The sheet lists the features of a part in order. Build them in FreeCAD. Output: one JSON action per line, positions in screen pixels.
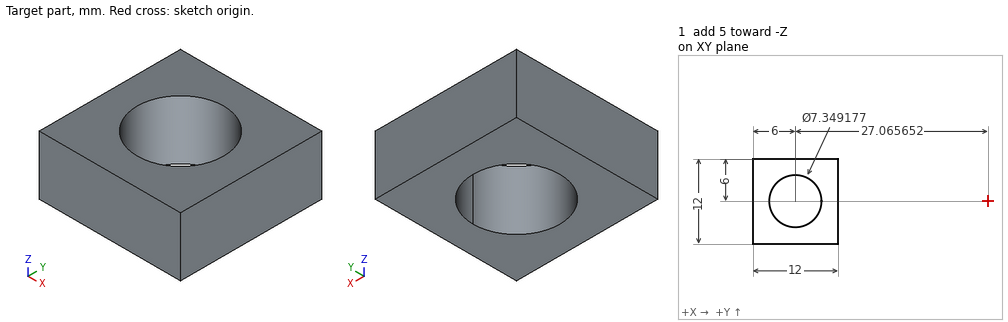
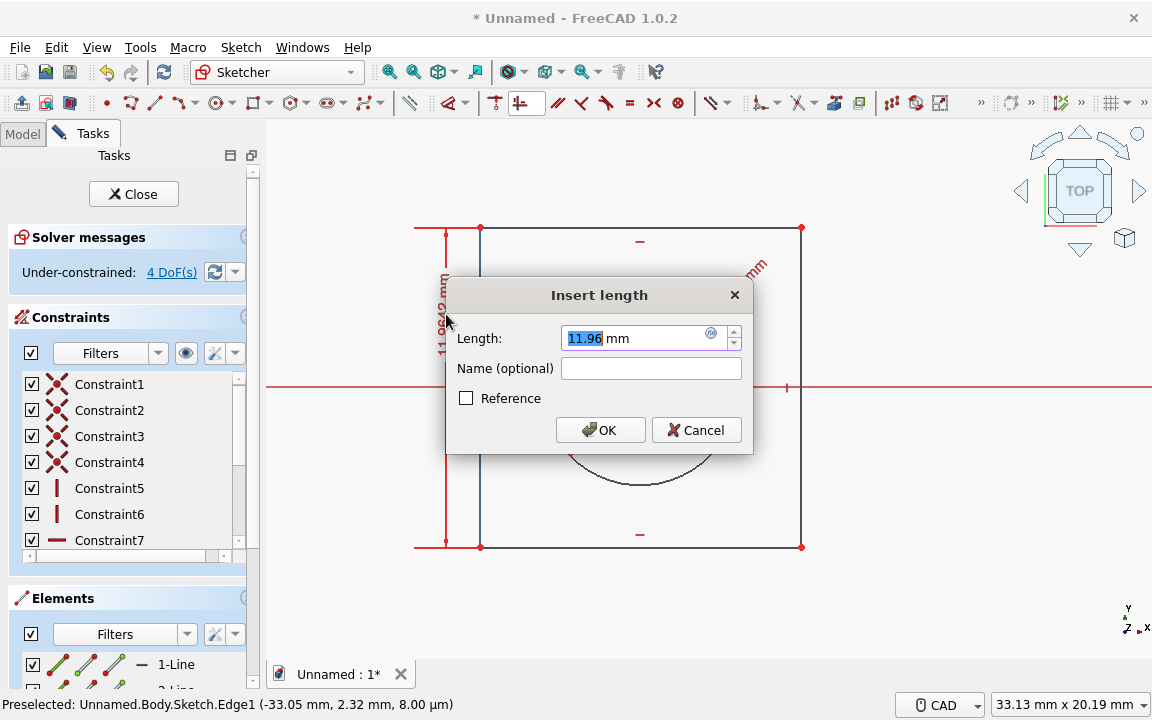
{"action": "type", "text": "12"}
{"action": "key", "text": "Return"}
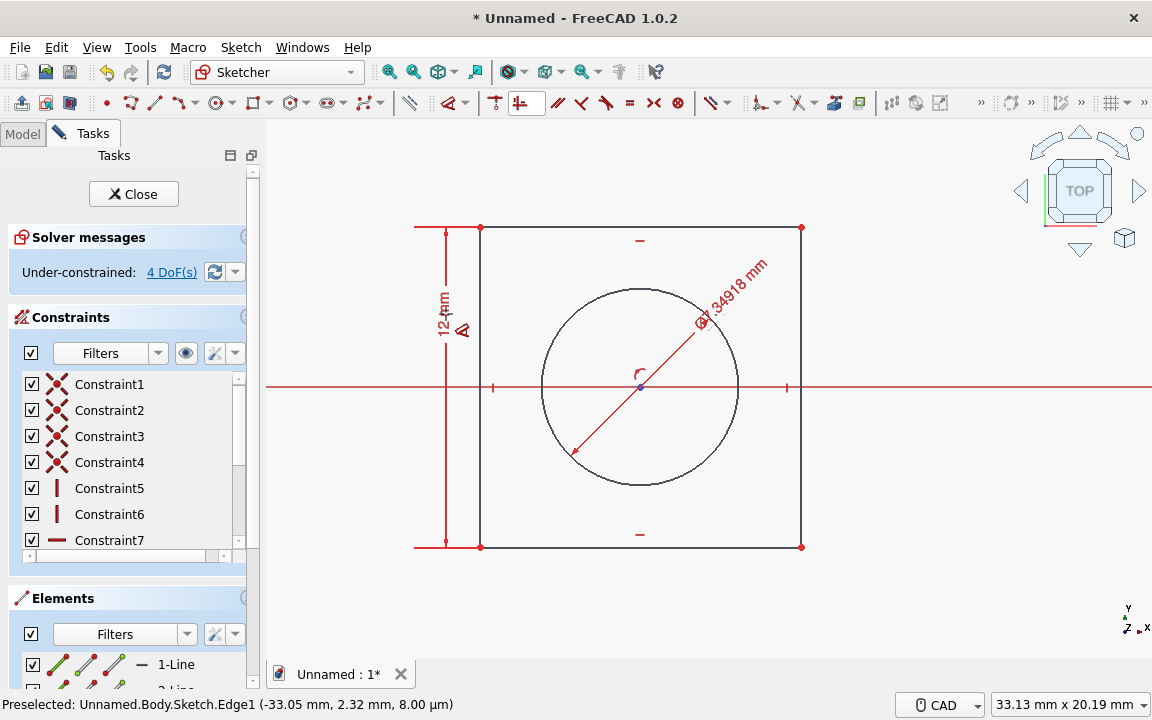
{"action": "left_click", "coordinate": [576, 548]}
{"action": "left_click", "coordinate": [641, 582]}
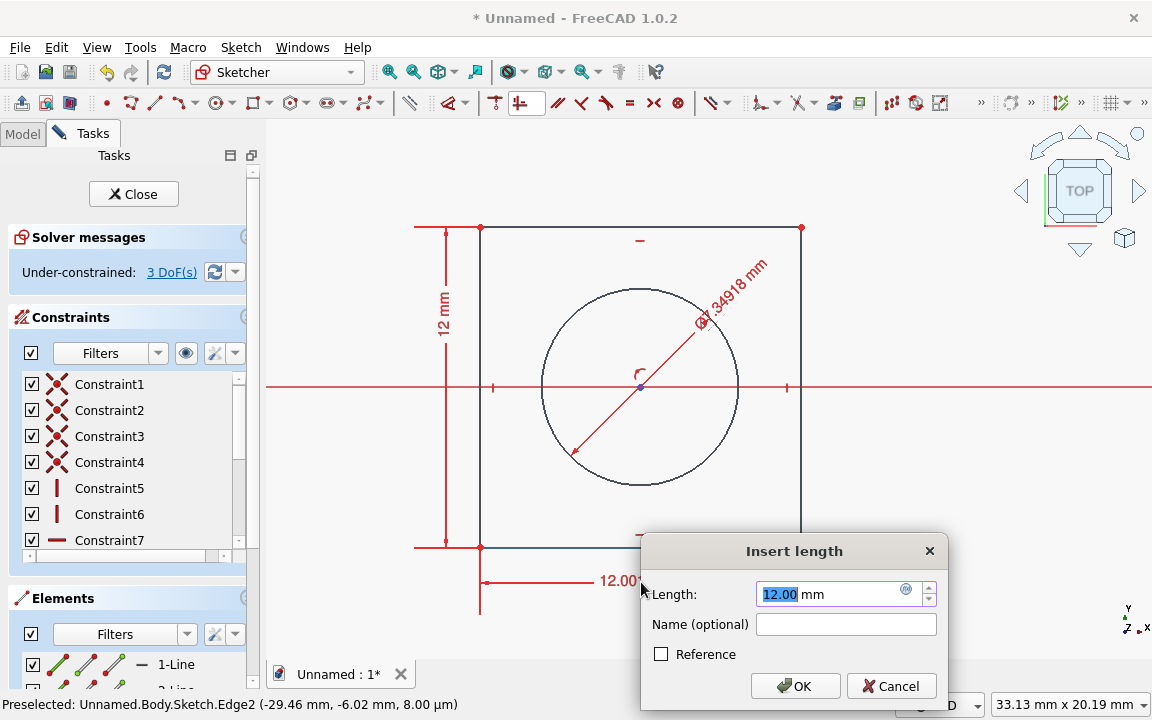
{"action": "type", "text": "12"}
{"action": "key", "text": "Return"}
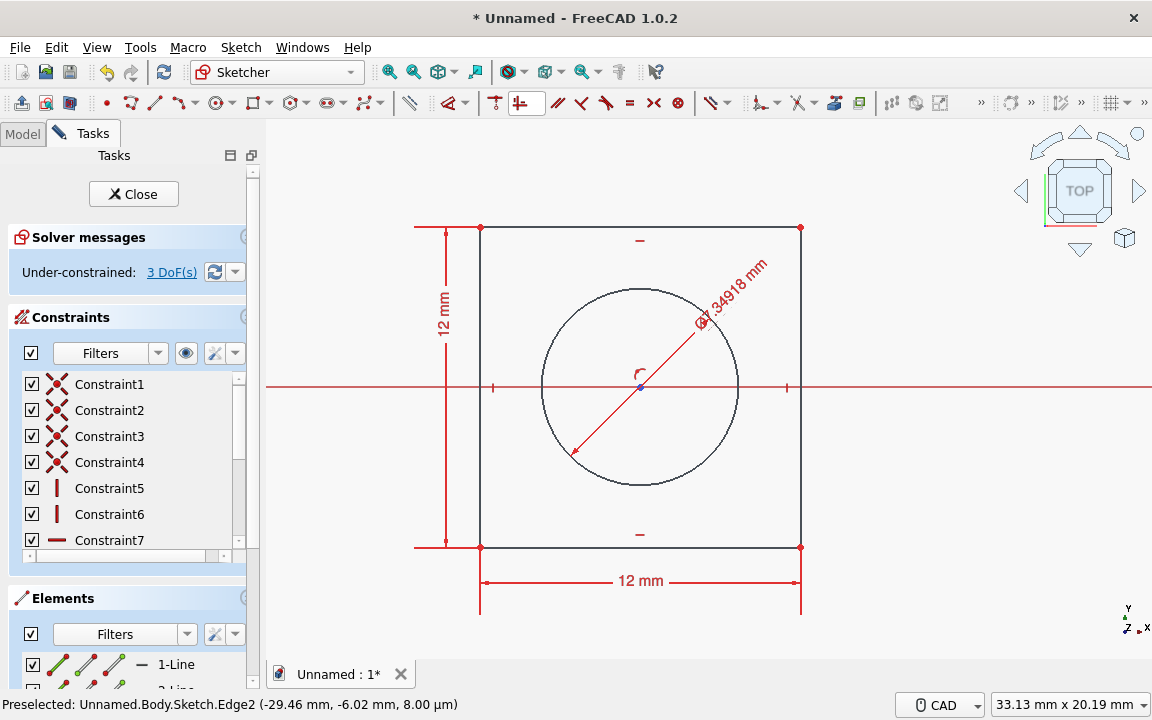
{"action": "left_click", "coordinate": [480, 227]}
{"action": "left_click", "coordinate": [446, 270]}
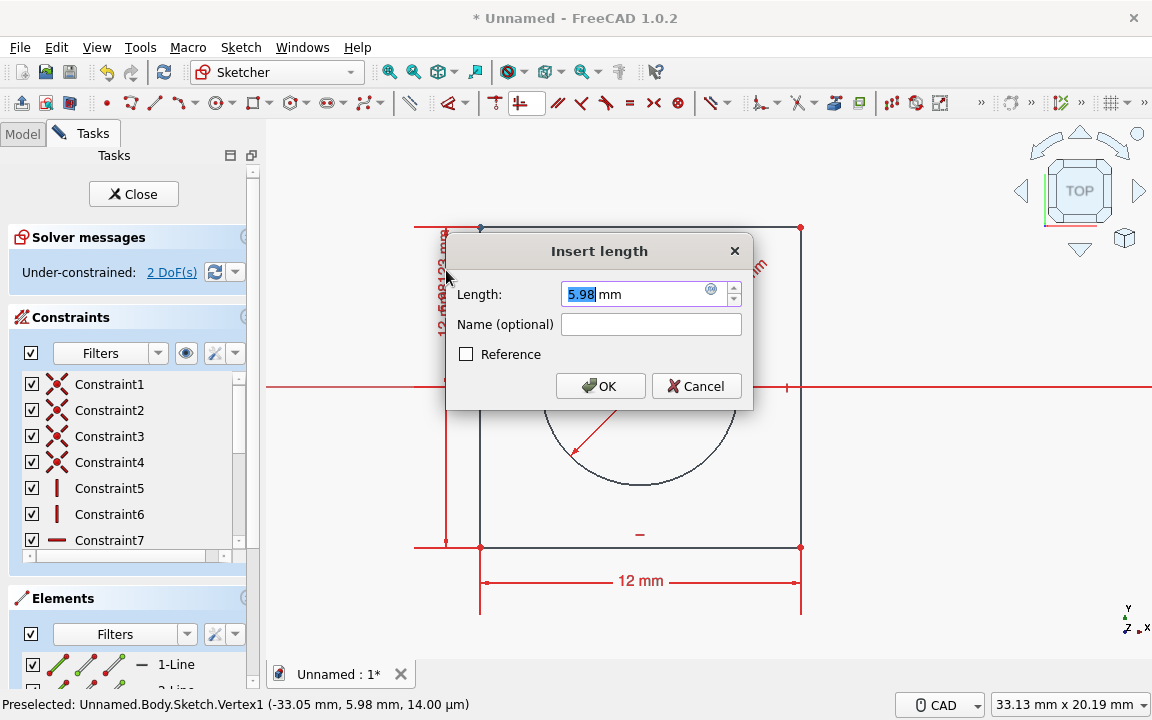
{"action": "type", "text": "6"}
{"action": "key", "text": "Return"}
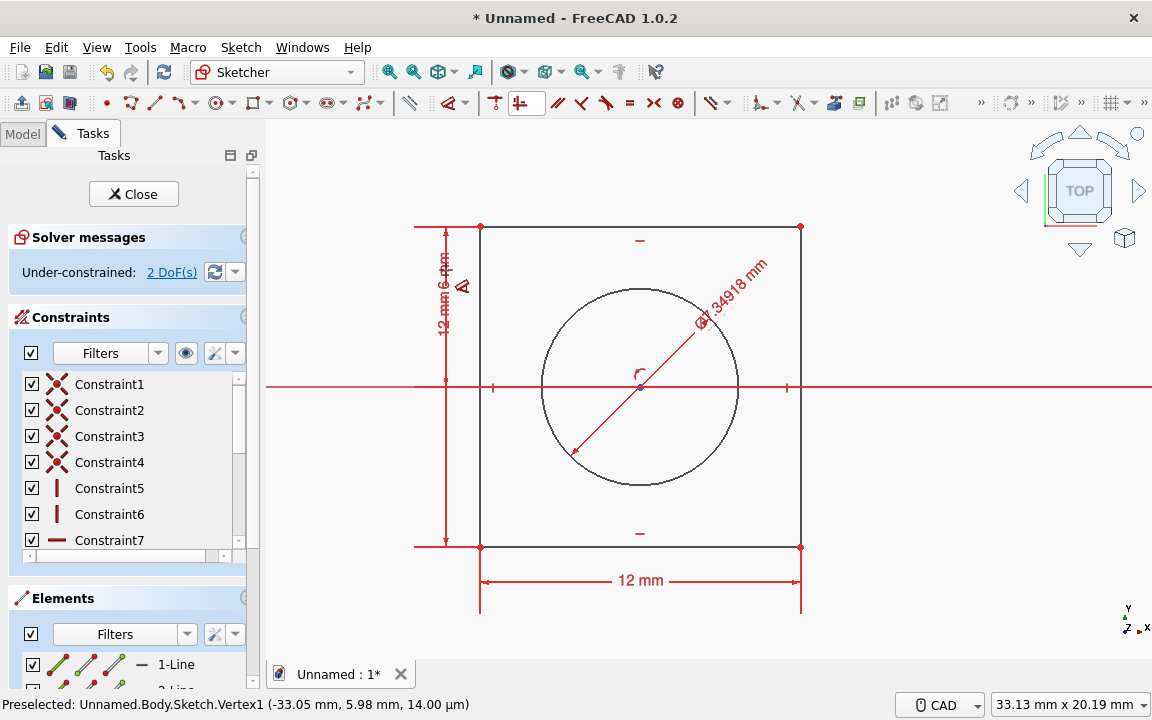
{"action": "left_click", "coordinate": [480, 227]}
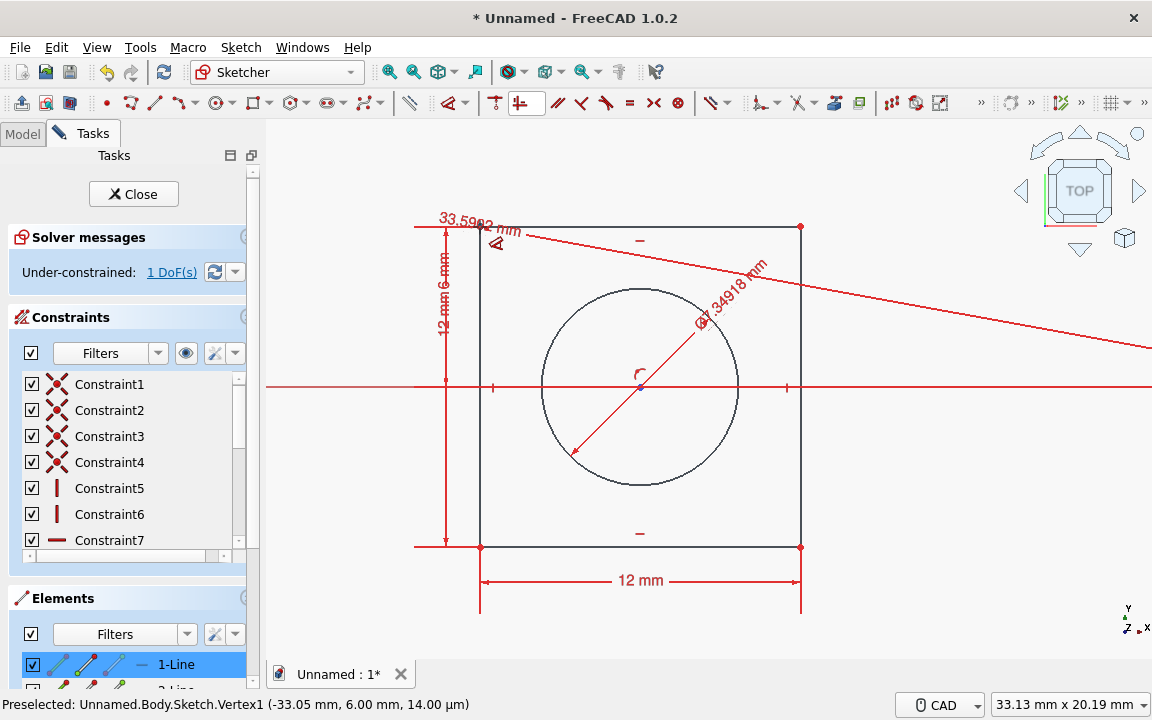
{"action": "left_click", "coordinate": [640, 387]}
{"action": "left_click", "coordinate": [560, 193]}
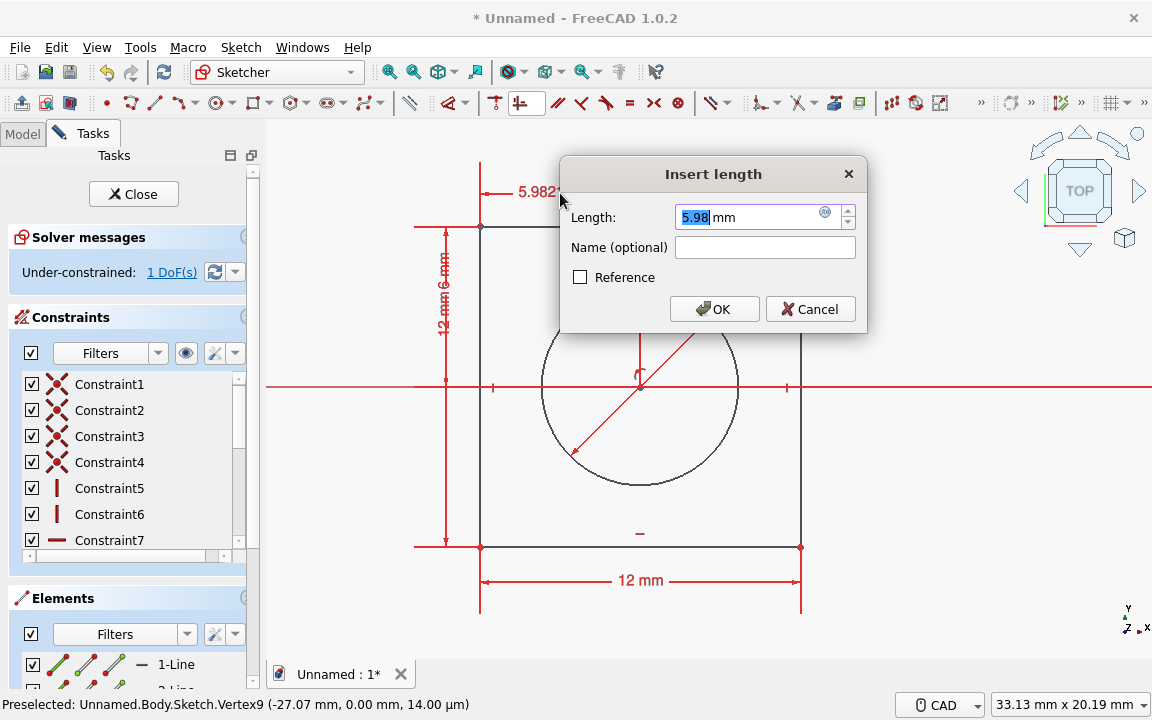
{"action": "type", "text": "6"}
{"action": "key", "text": "Return"}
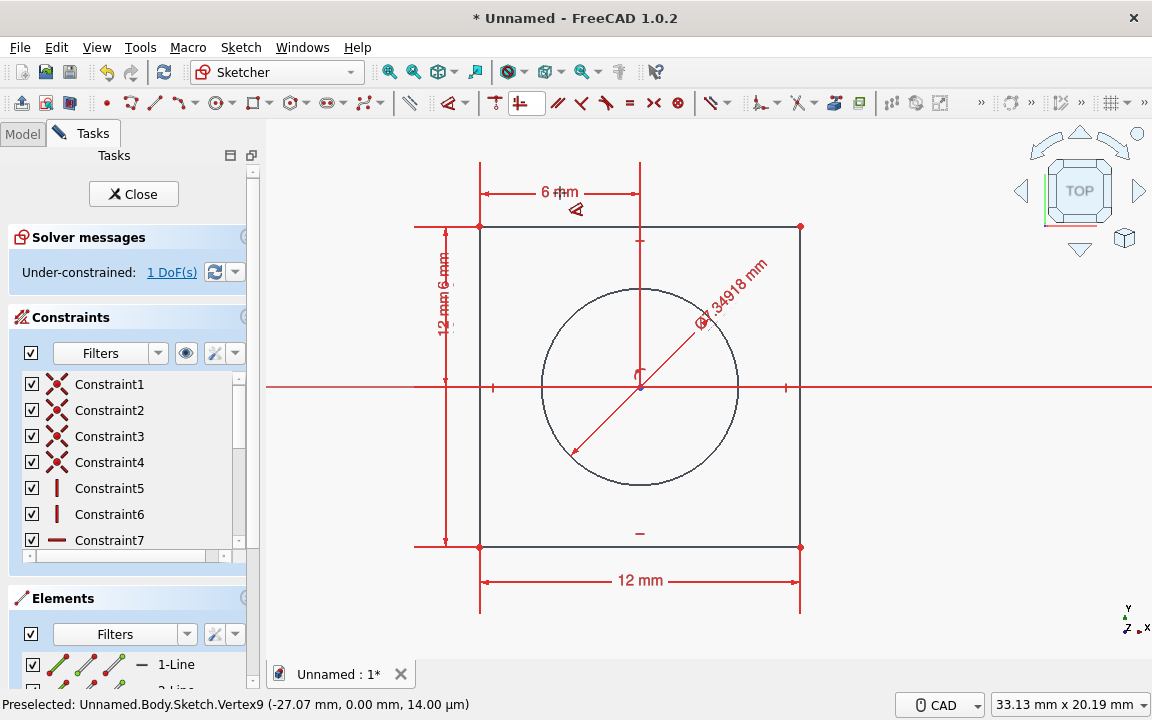
{"action": "left_click", "coordinate": [640, 387]}
{"action": "left_click", "coordinate": [813, 421]}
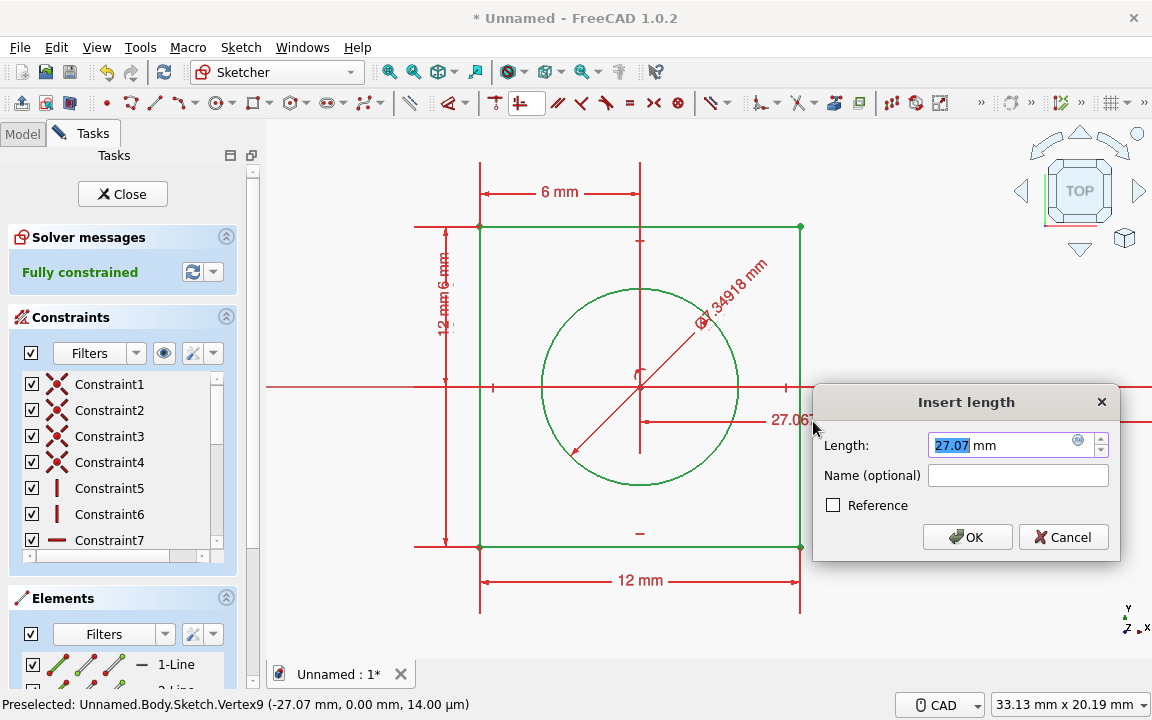
{"action": "type", "text": "27.065652"}
{"action": "key", "text": "Return"}
{"action": "key", "text": "Escape"}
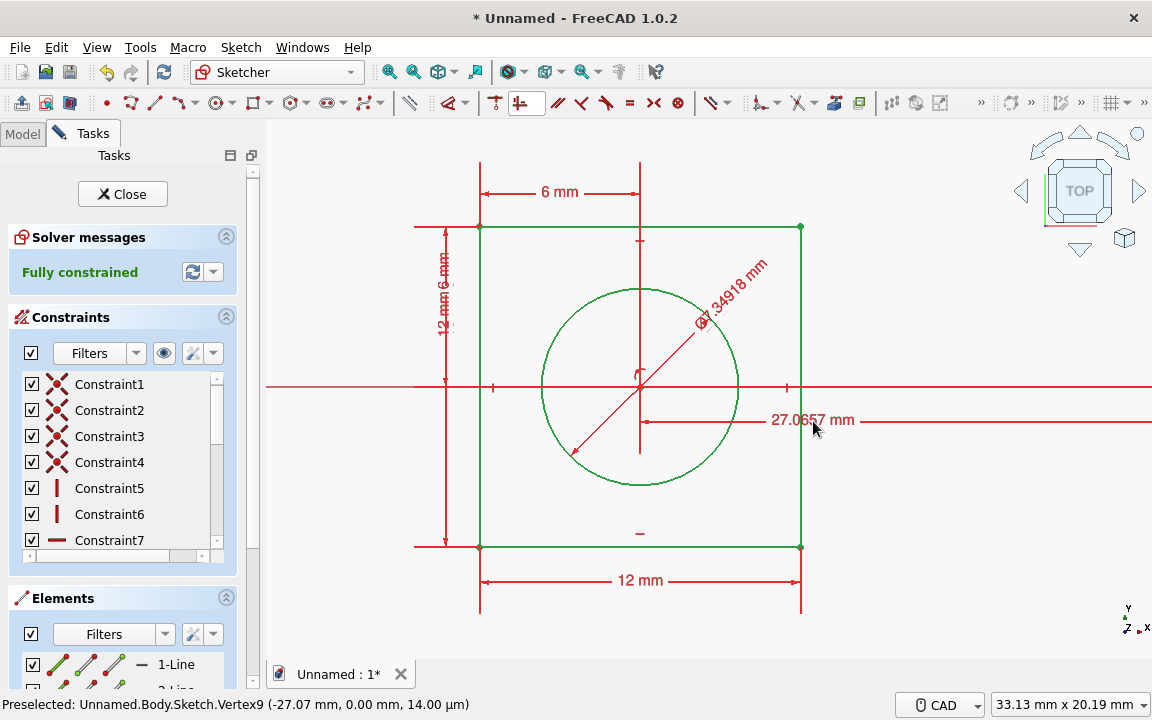
{"action": "left_click", "coordinate": [123, 194]}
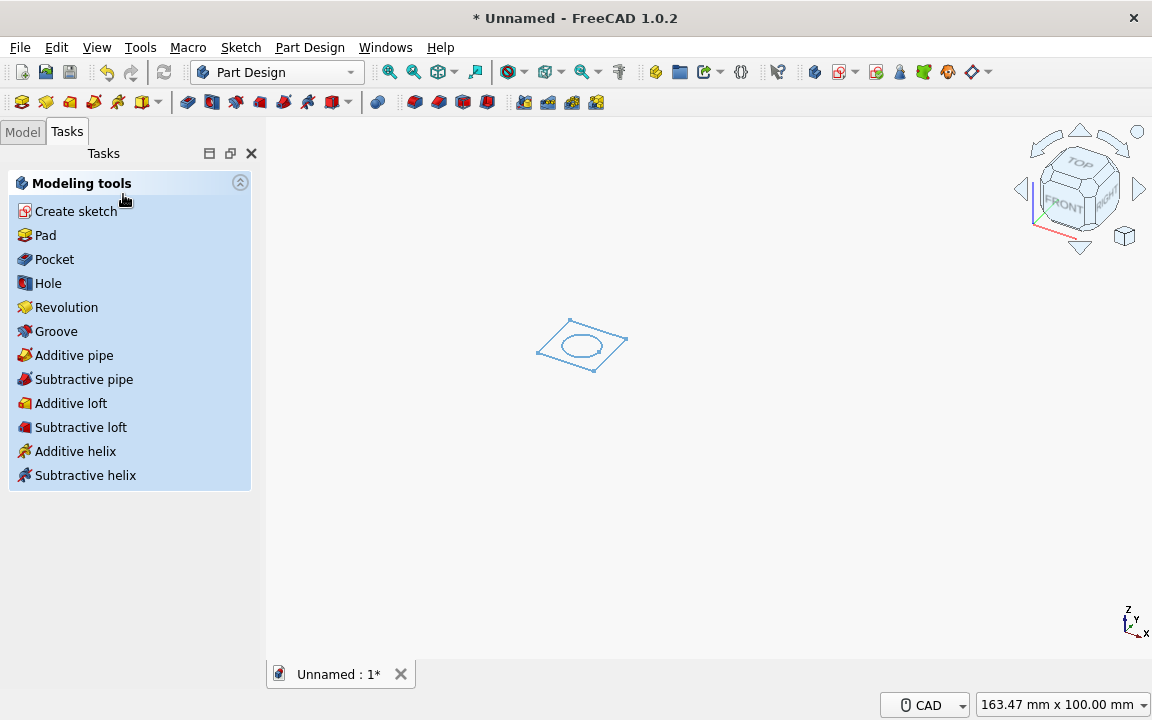
{"action": "left_click", "coordinate": [22, 102]}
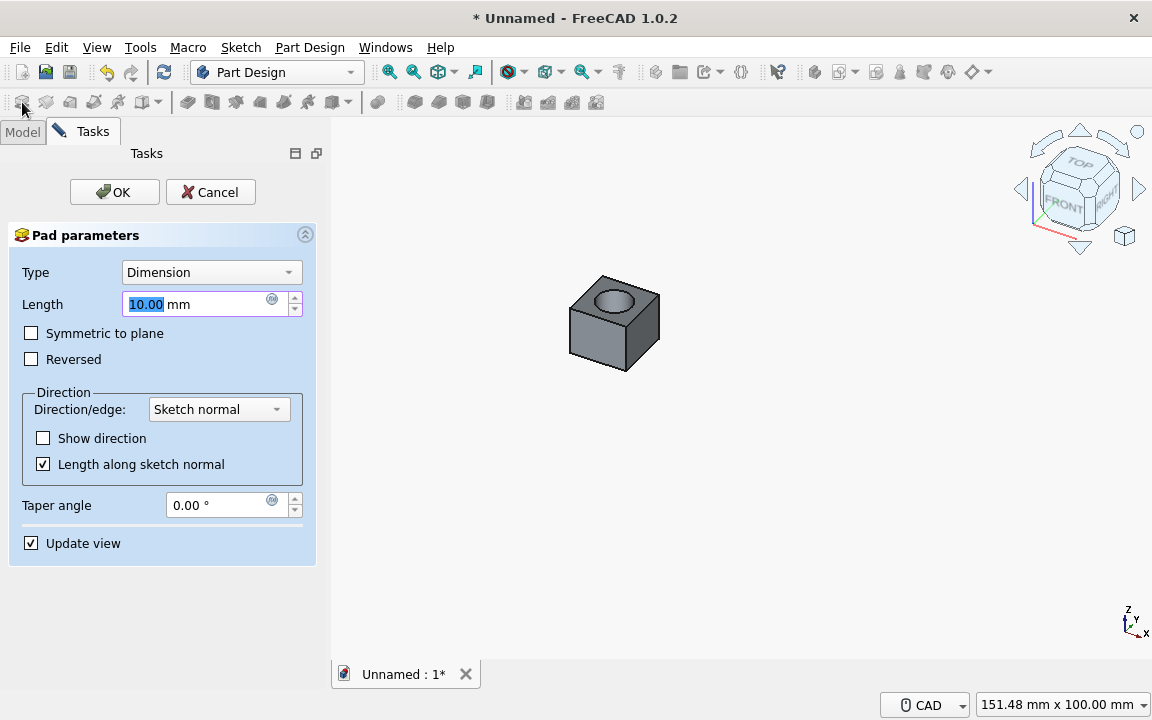
{"action": "type", "text": "5"}
{"action": "key", "text": "Tab"}